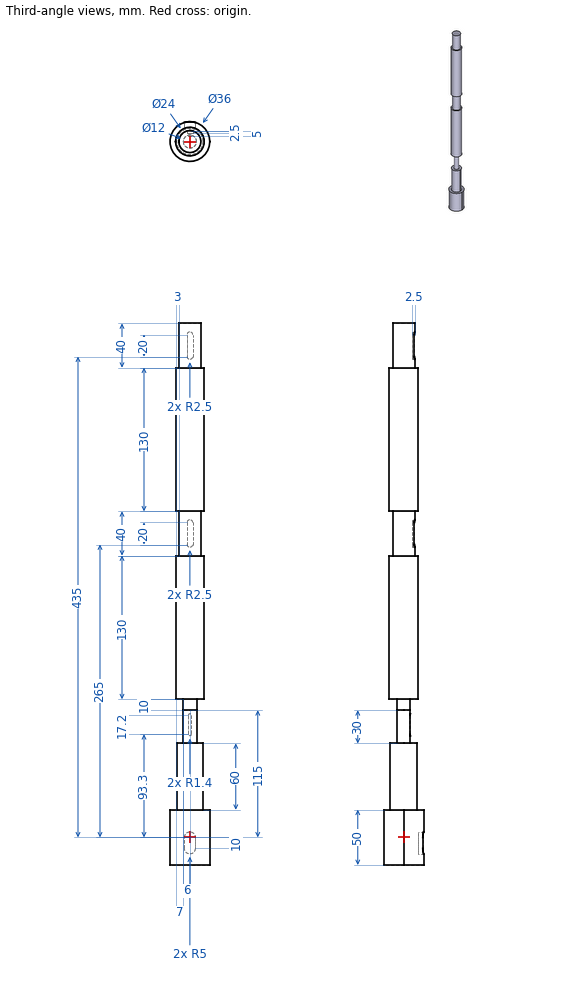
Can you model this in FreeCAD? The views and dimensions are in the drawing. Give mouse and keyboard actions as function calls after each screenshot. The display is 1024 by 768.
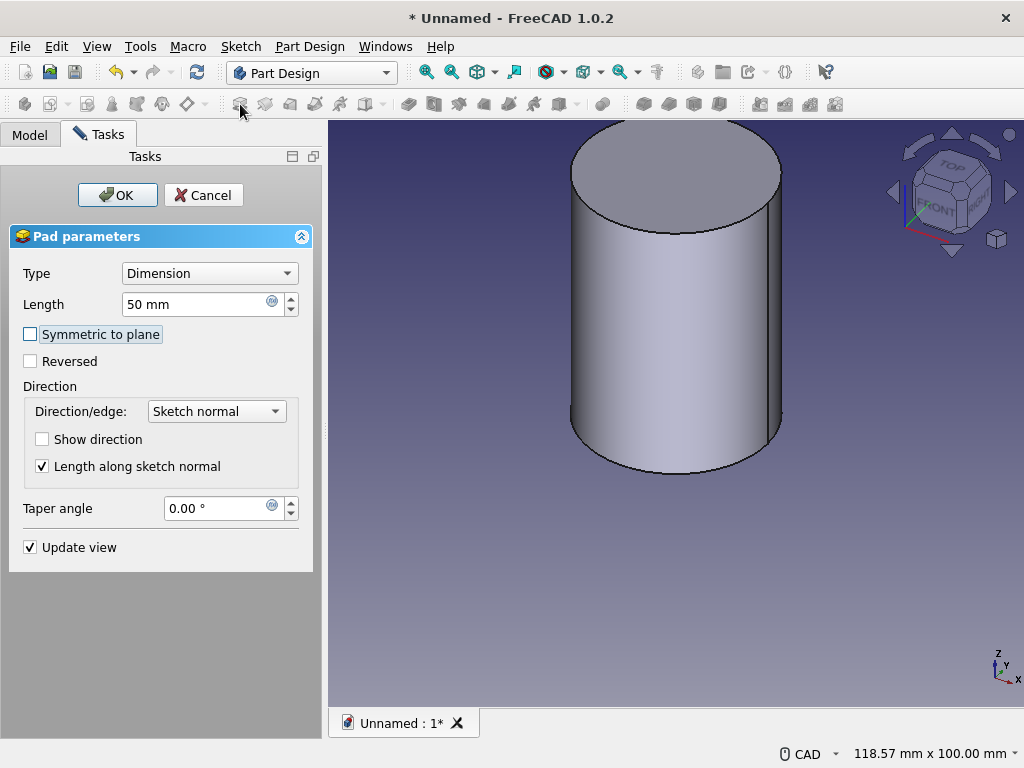
click(31, 334)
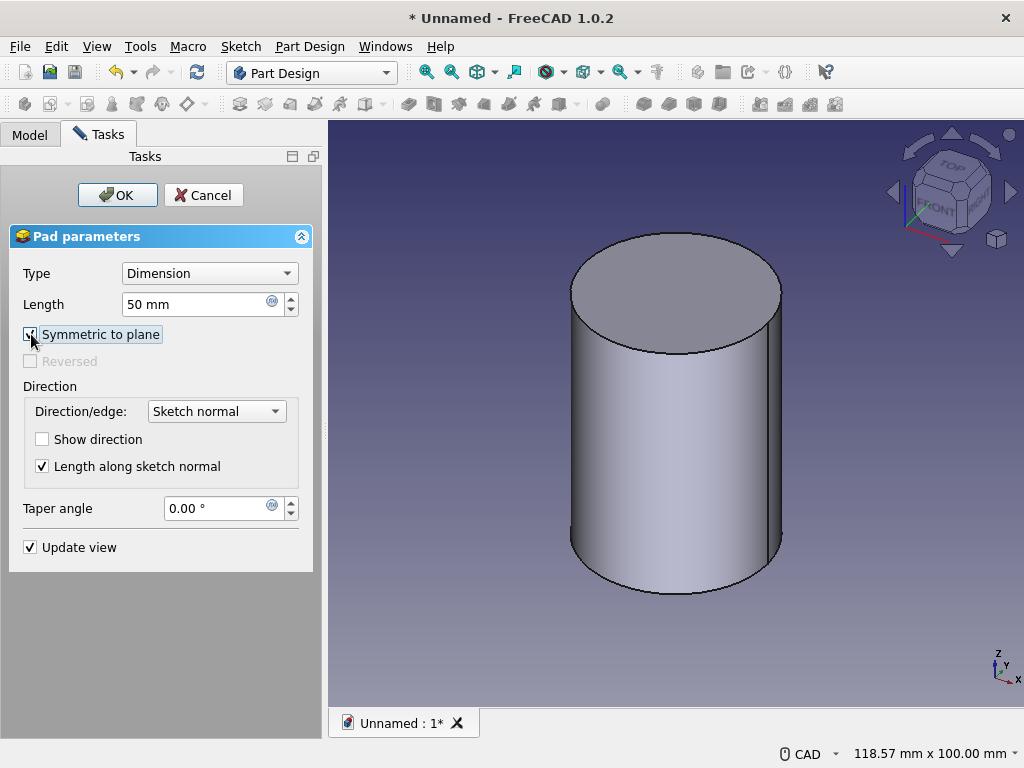
click(118, 195)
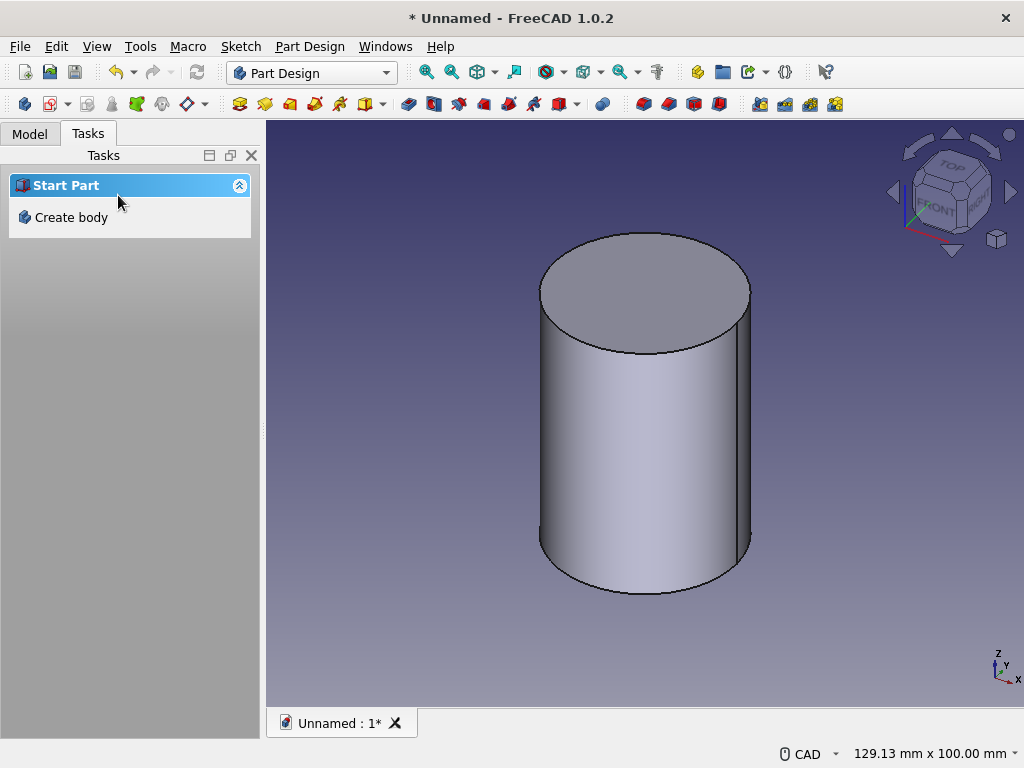
click(645, 292)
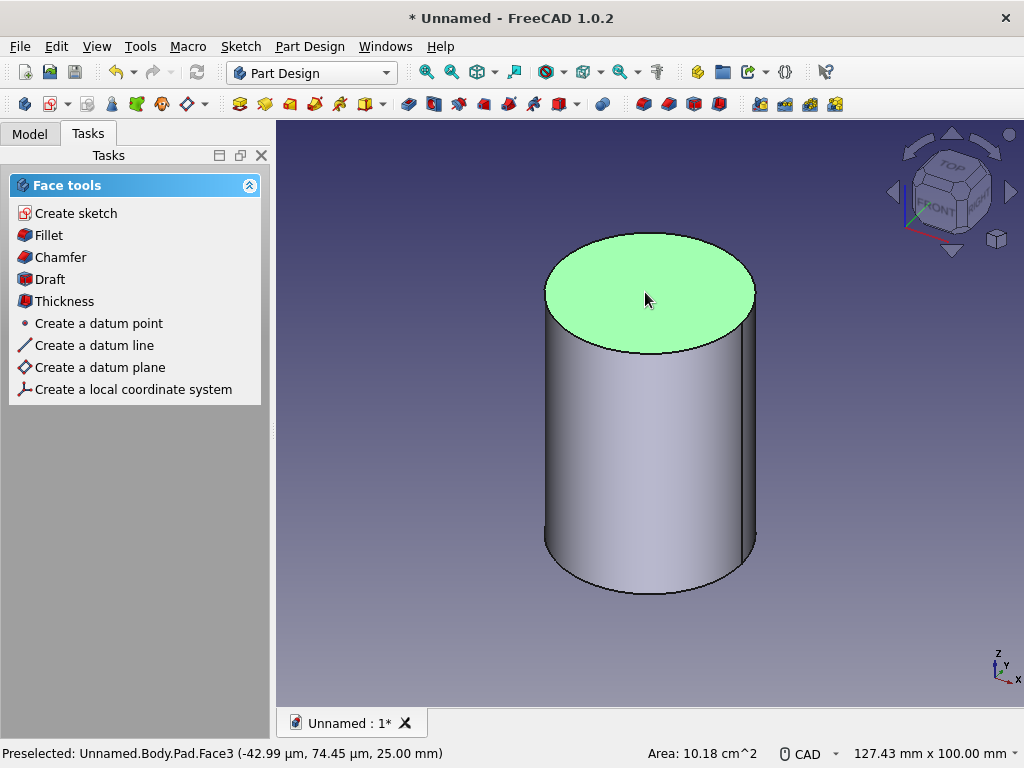
click(50, 104)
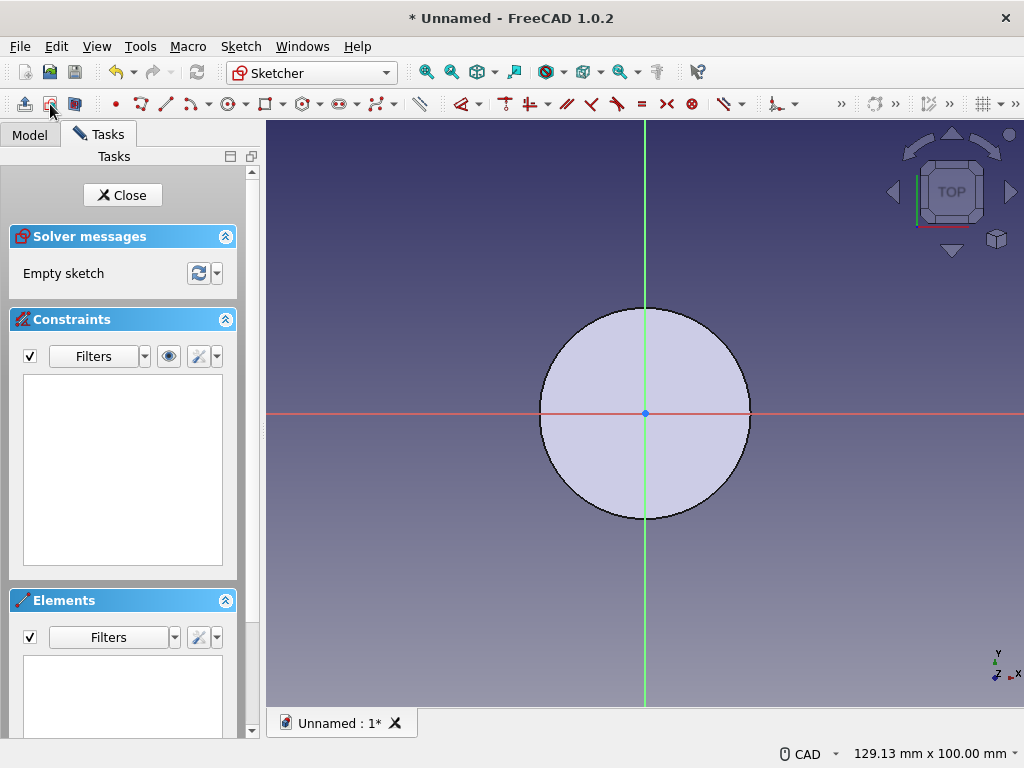
scroll(685, 414, up, 5)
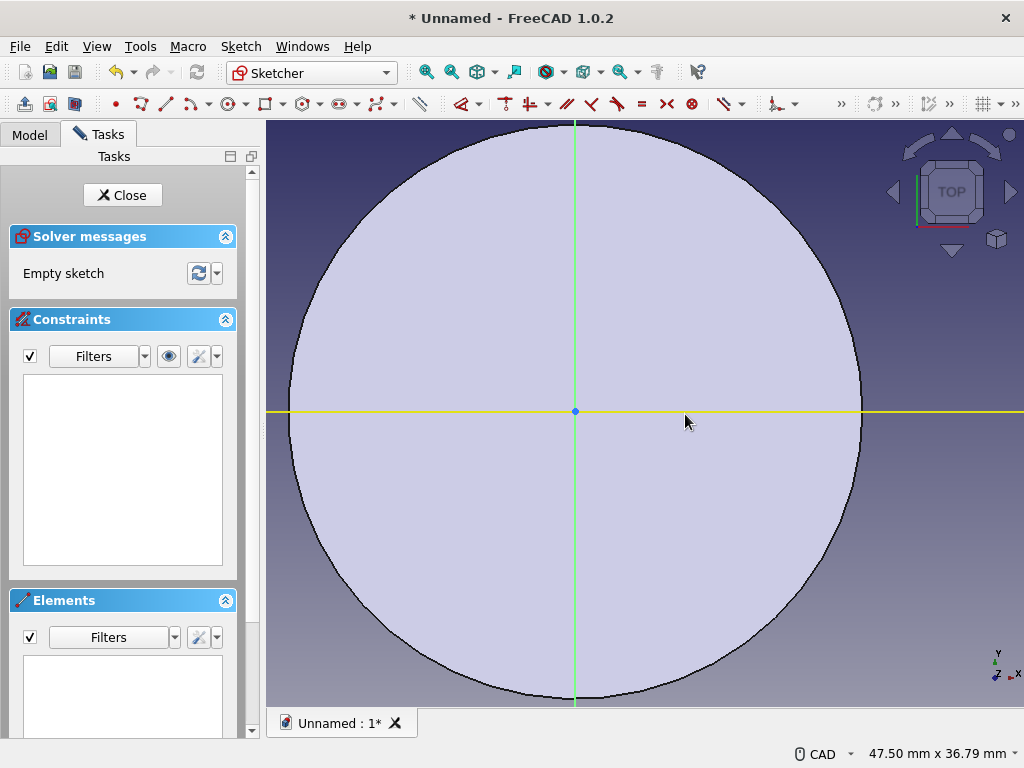
click(228, 104)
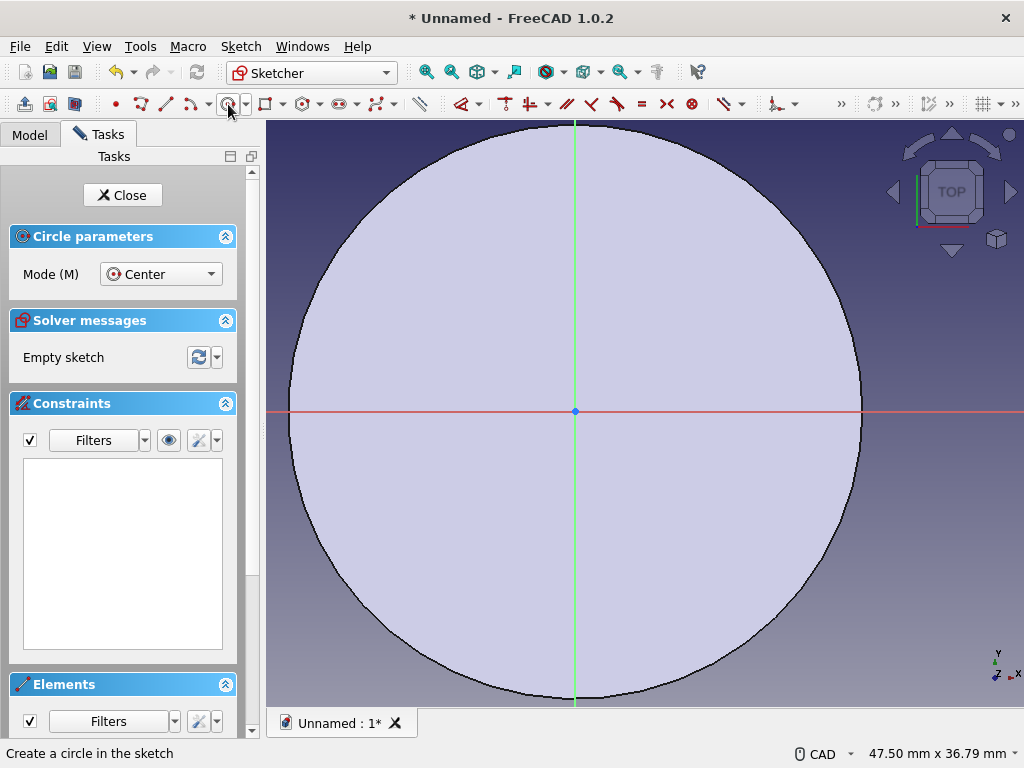
click(575, 412)
click(711, 276)
key(Escape)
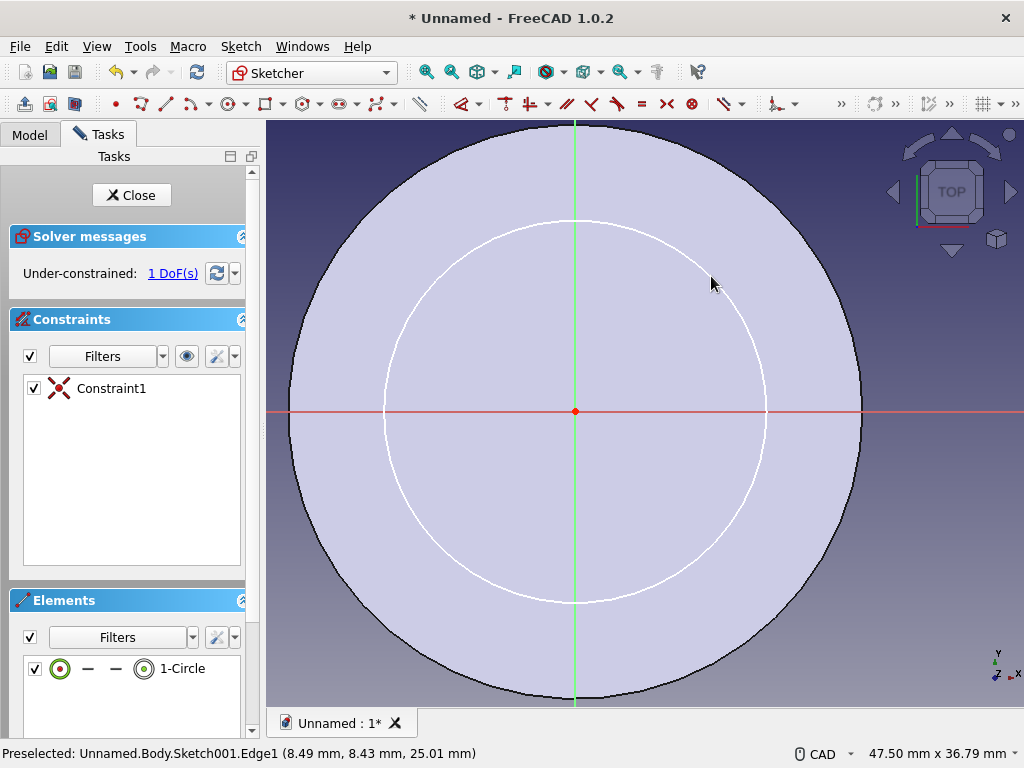
click(460, 104)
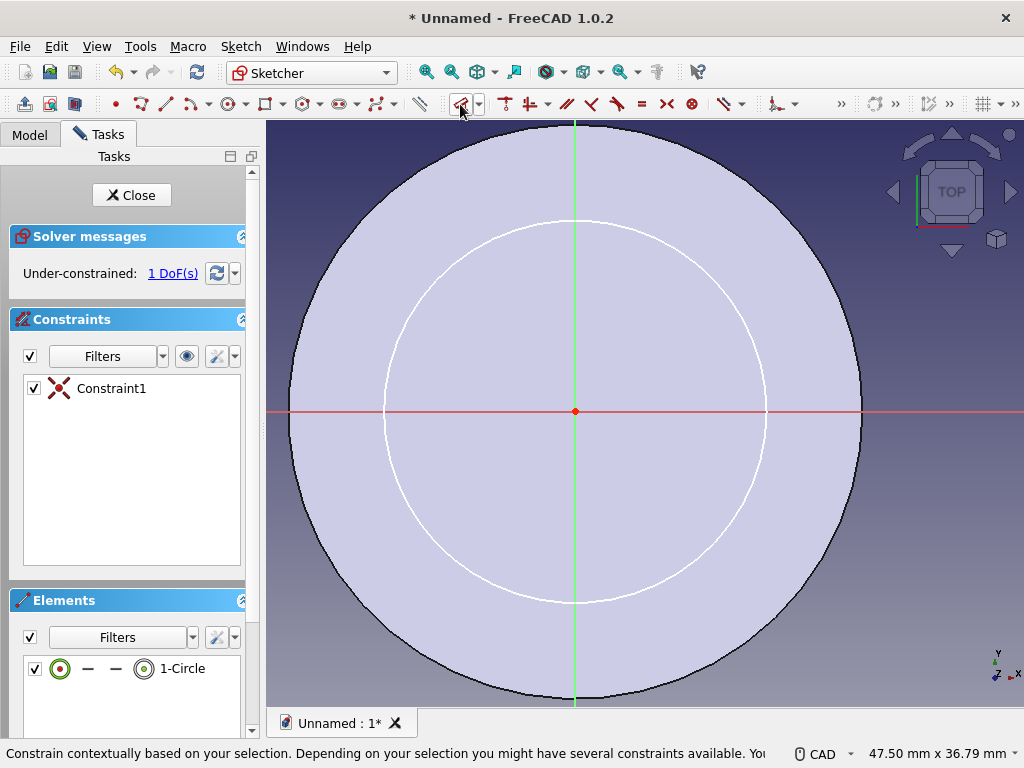
click(710, 276)
click(733, 253)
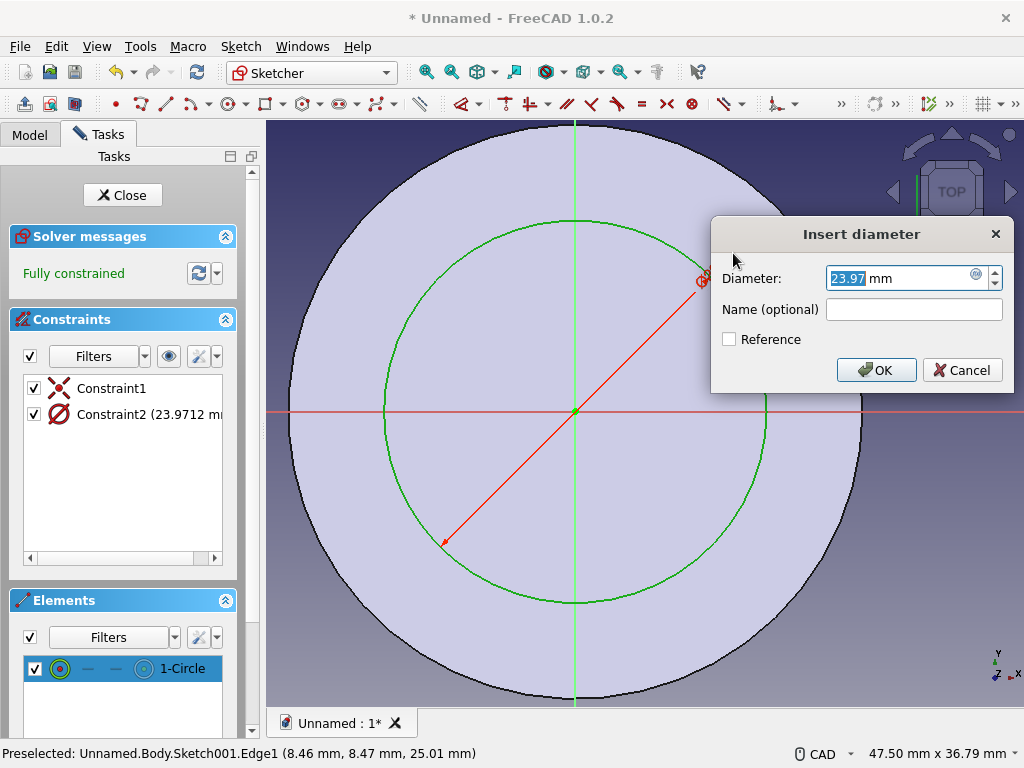
text(24)
key(Return)
key(Escape)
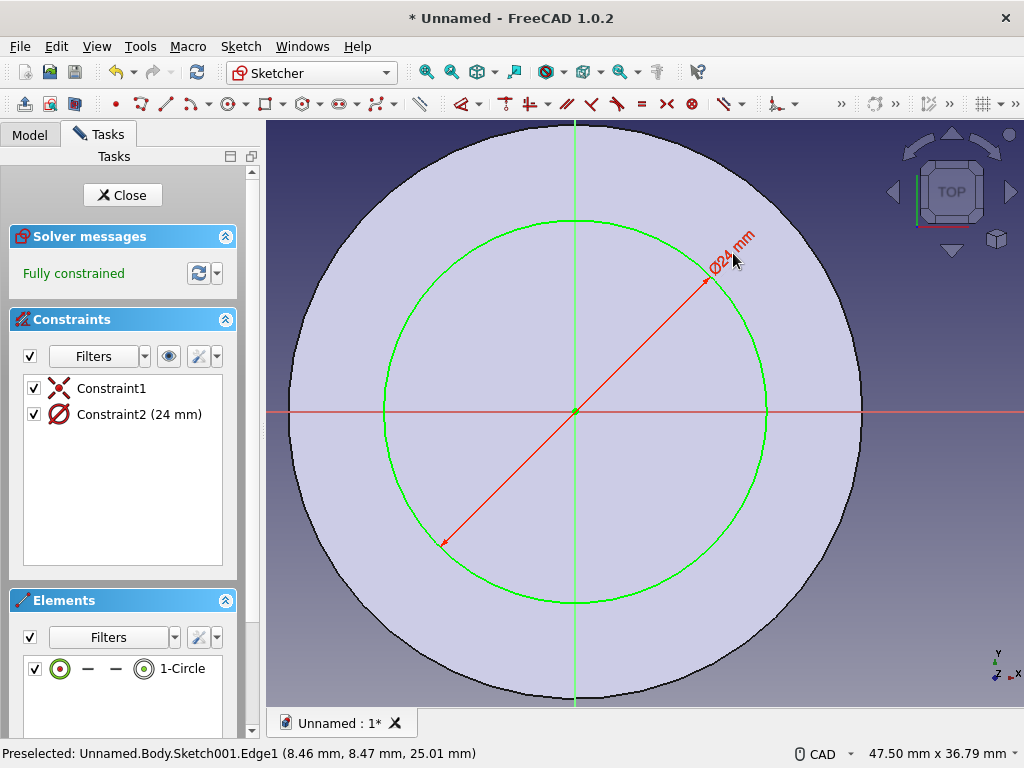
click(123, 195)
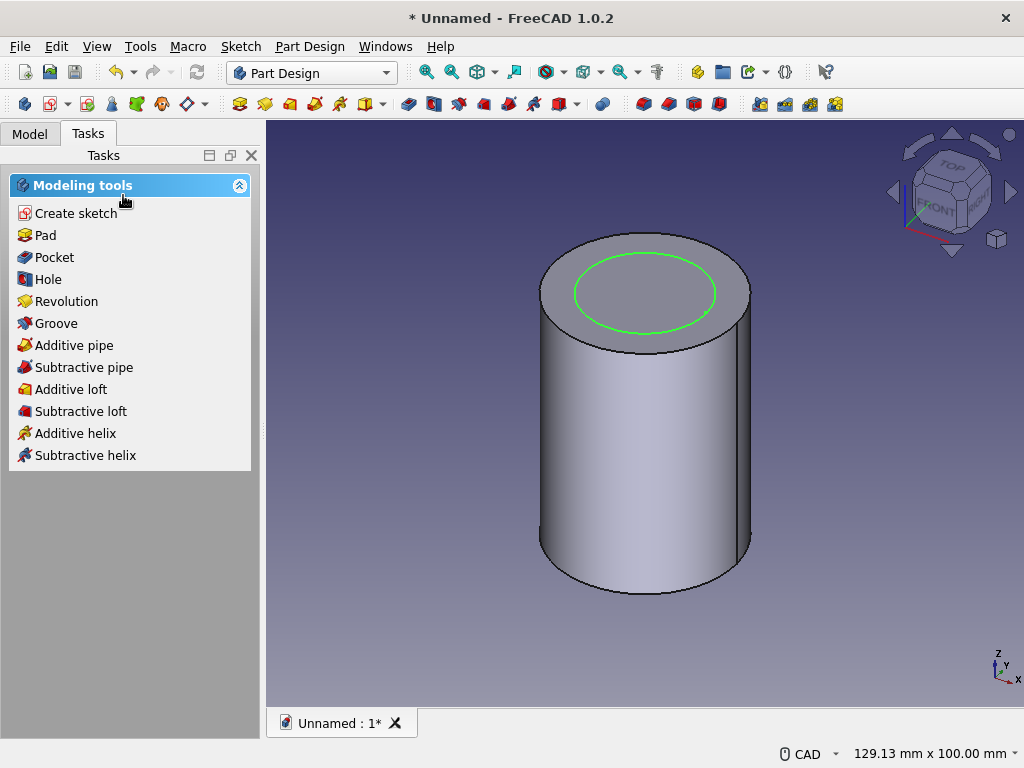
click(240, 104)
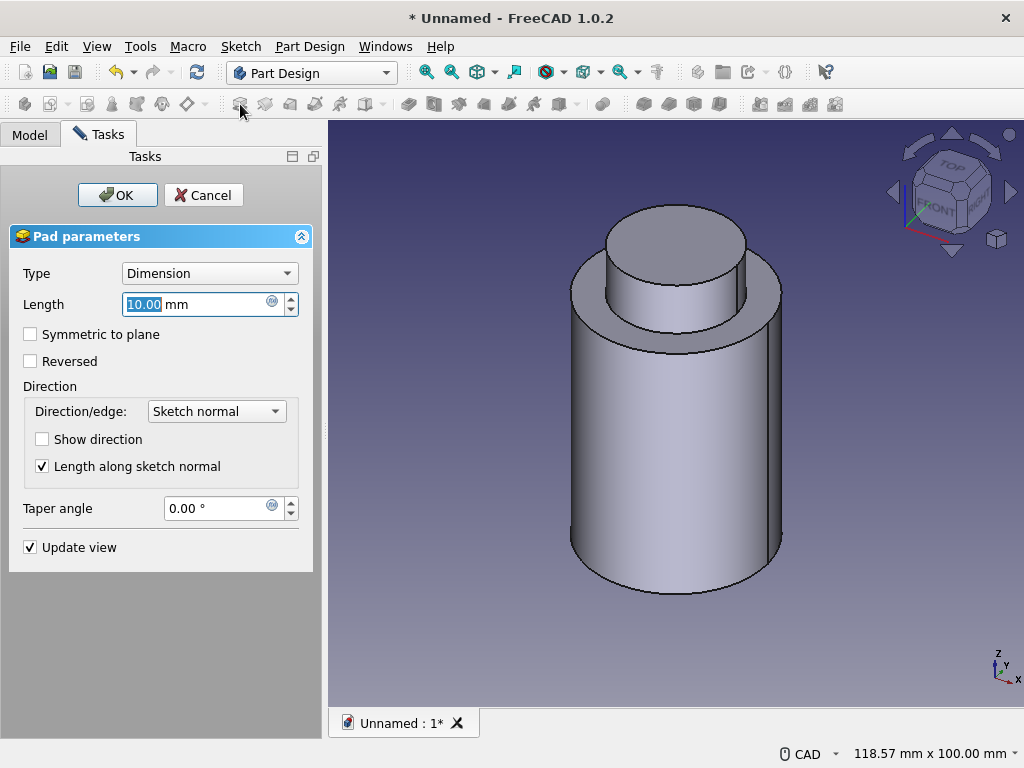
text(60)
key(Tab)